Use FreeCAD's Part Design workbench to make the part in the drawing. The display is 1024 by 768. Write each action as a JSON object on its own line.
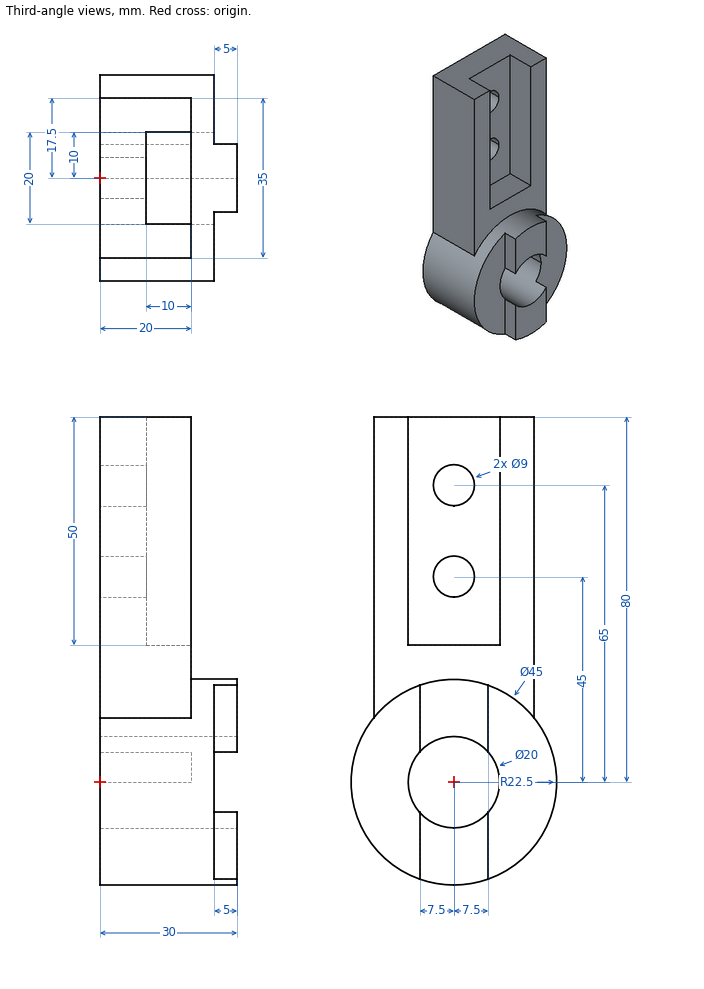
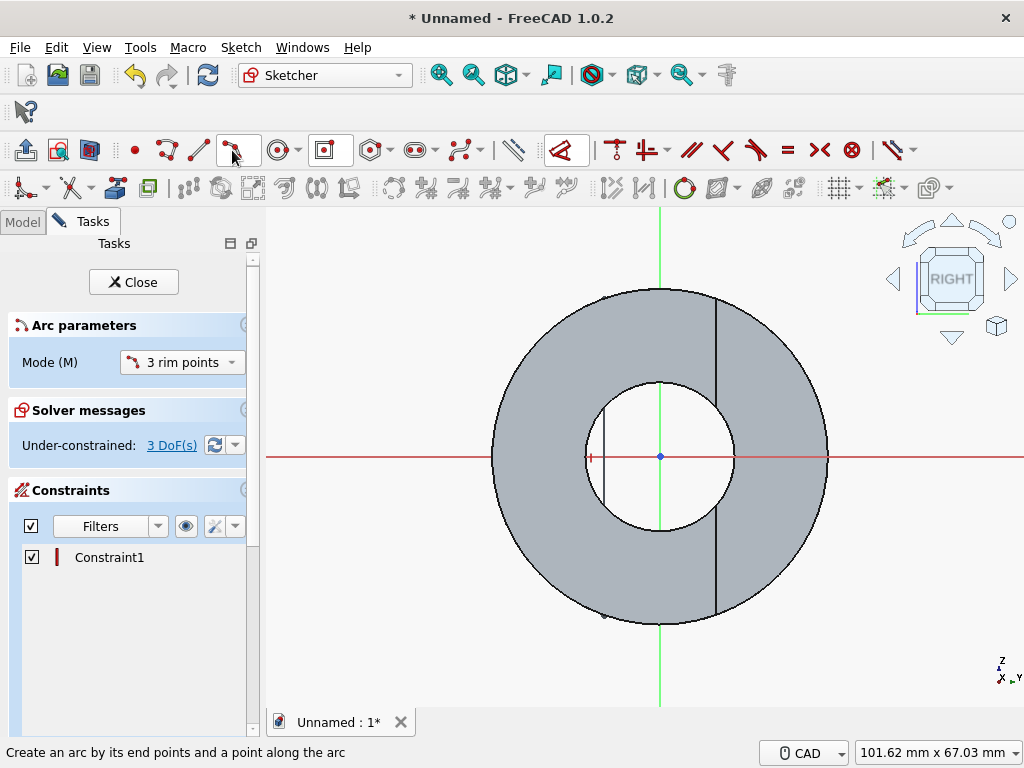
{"action": "left_click", "coordinate": [604, 300]}
{"action": "left_click", "coordinate": [604, 616]}
{"action": "left_click", "coordinate": [497, 416]}
{"action": "key", "text": "Escape"}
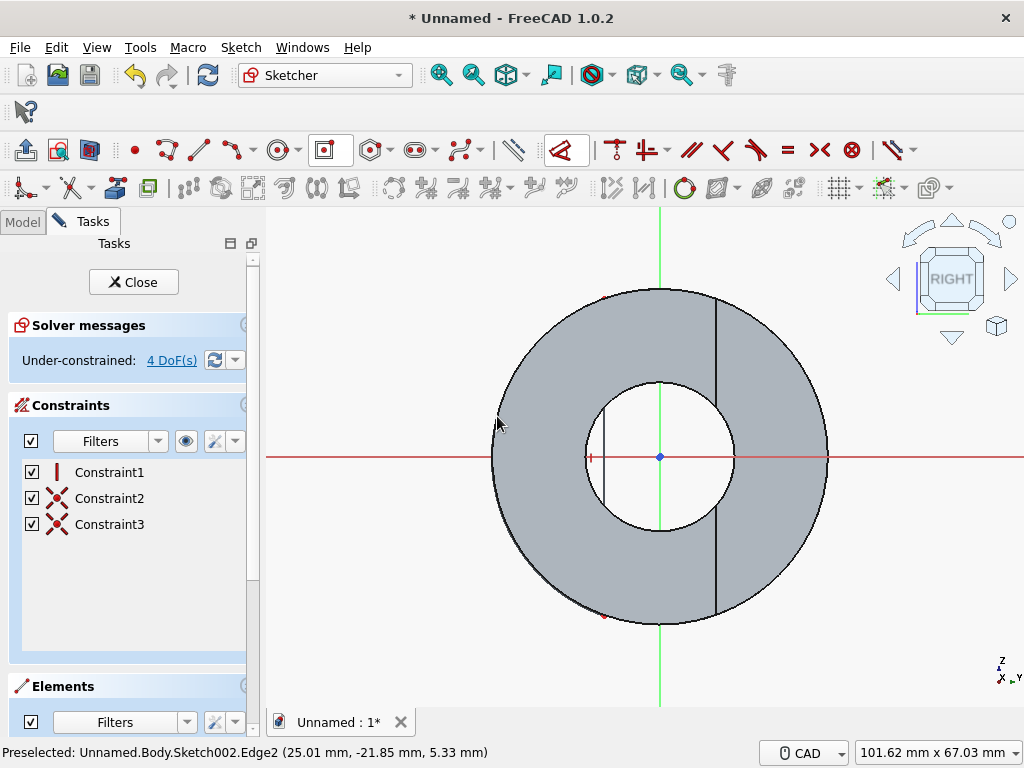
{"action": "left_click_drag", "start_coordinate": [649, 447], "coordinate": [670, 468]}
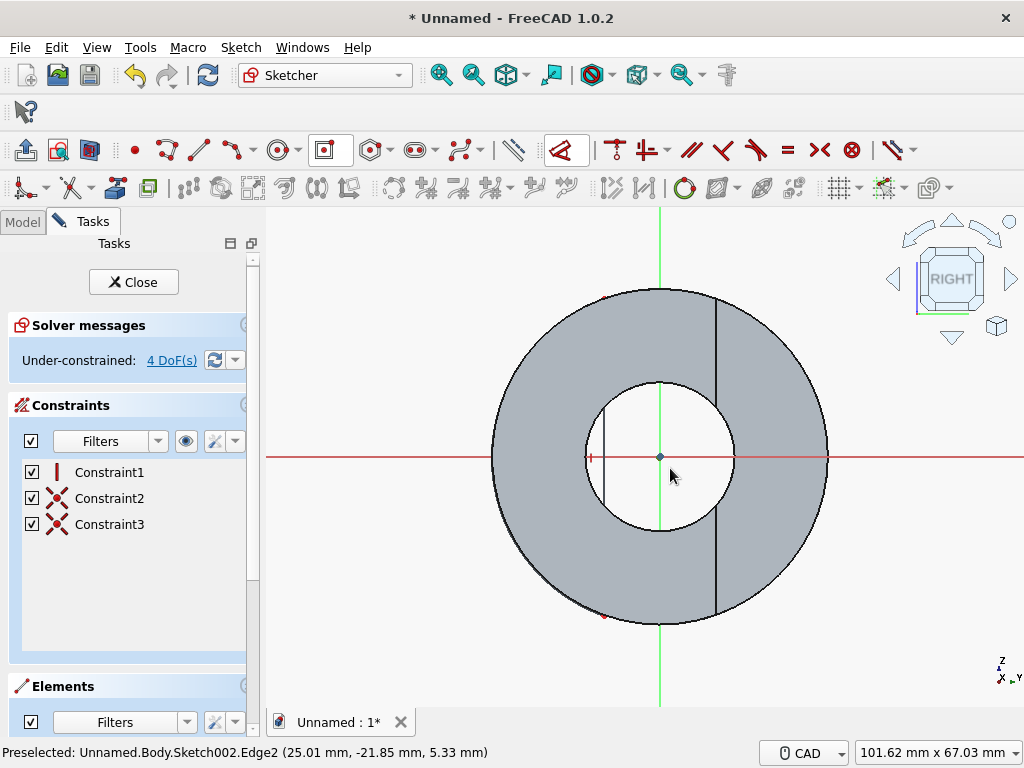
{"action": "left_click", "coordinate": [616, 150]}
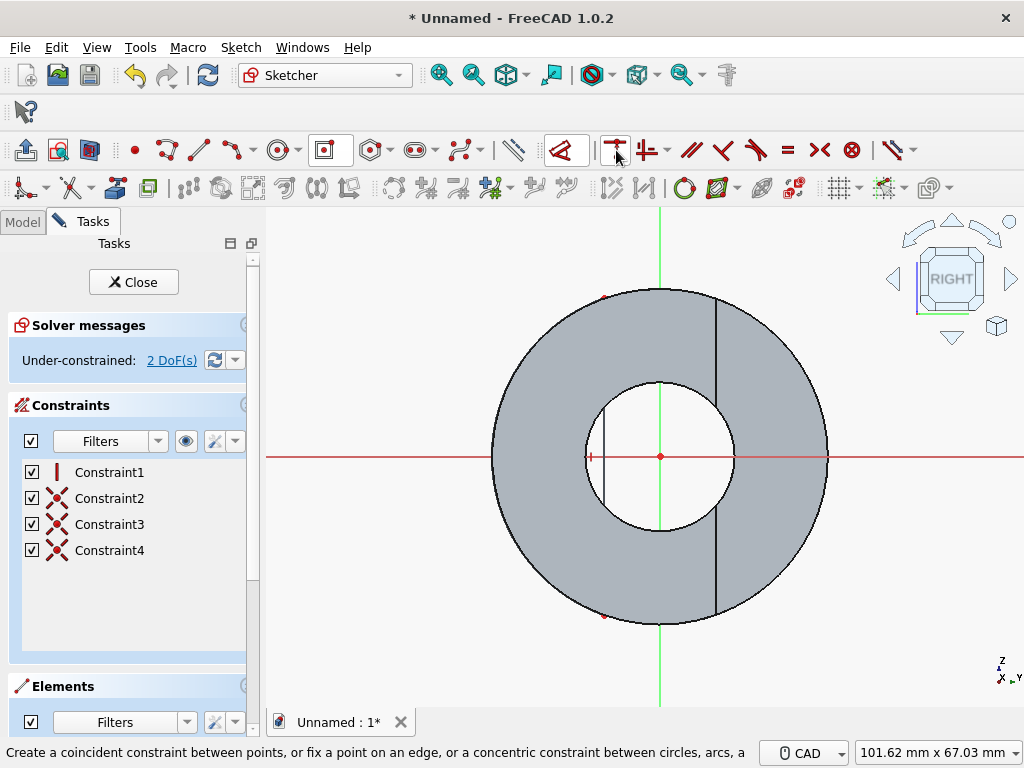
{"action": "left_click", "coordinate": [512, 377]}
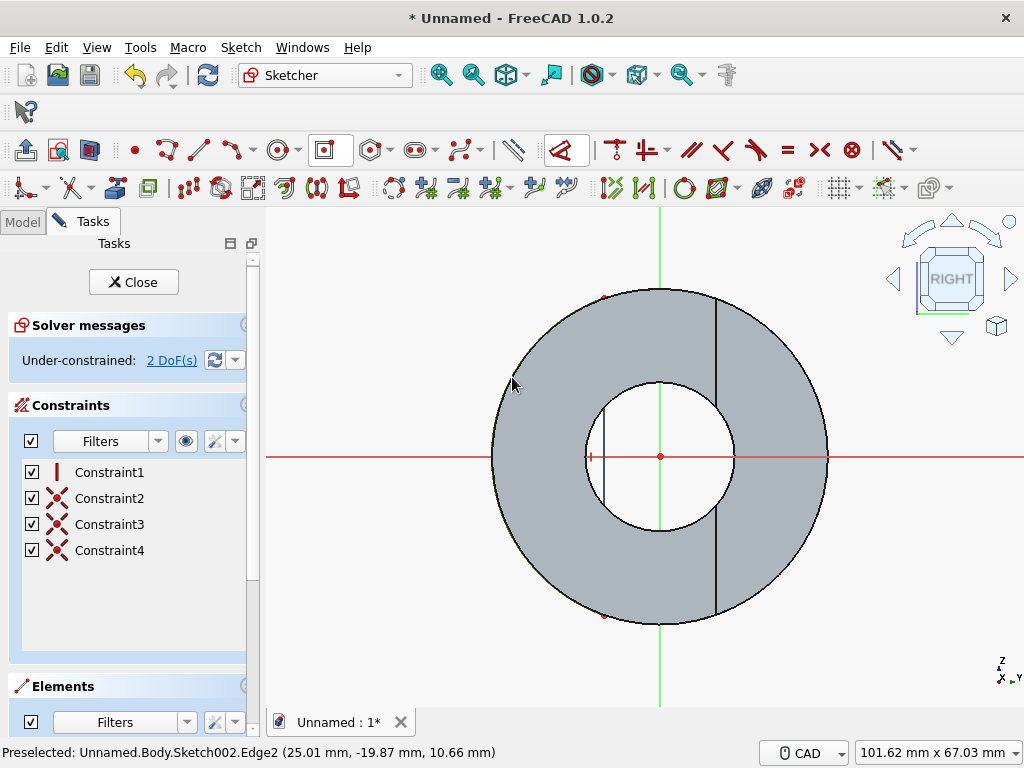
{"action": "key", "text": "k r"}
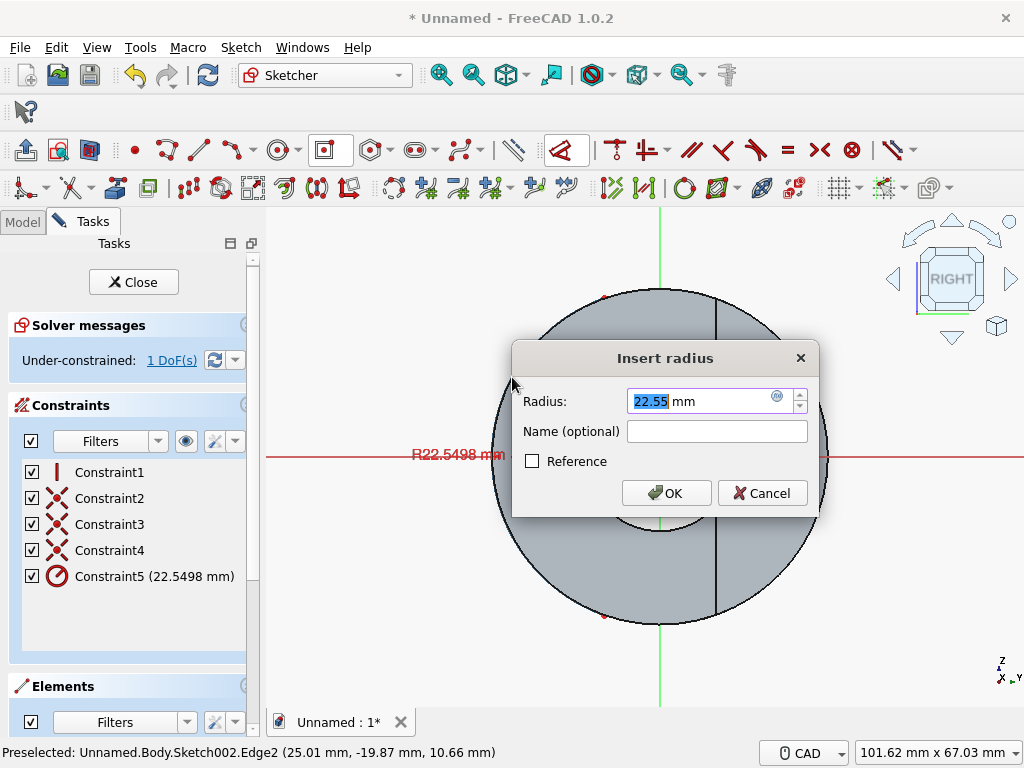
{"action": "type", "text": "22.5"}
{"action": "key", "text": "Return"}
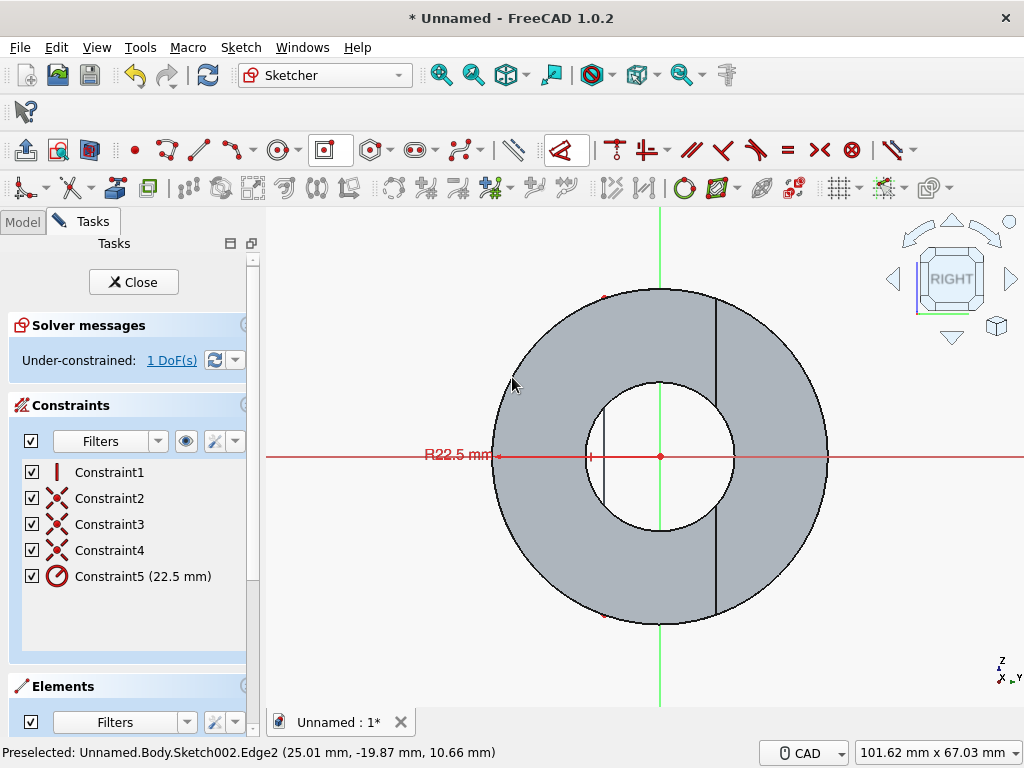
{"action": "left_click", "coordinate": [604, 615]}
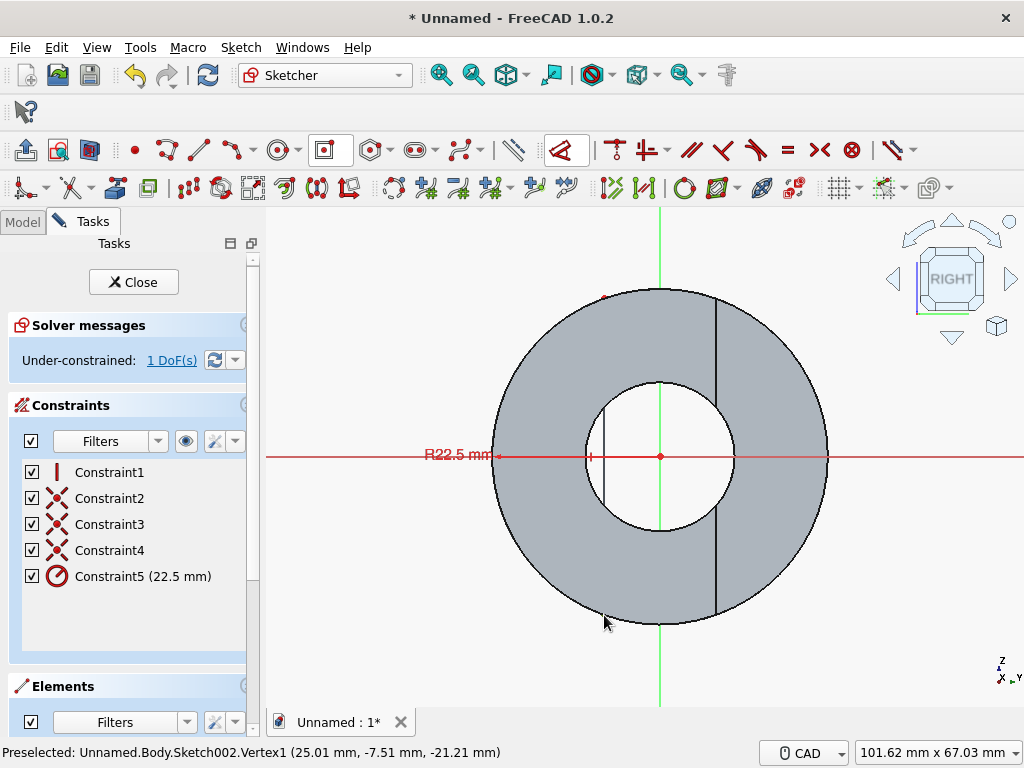
{"action": "left_click", "coordinate": [584, 150]}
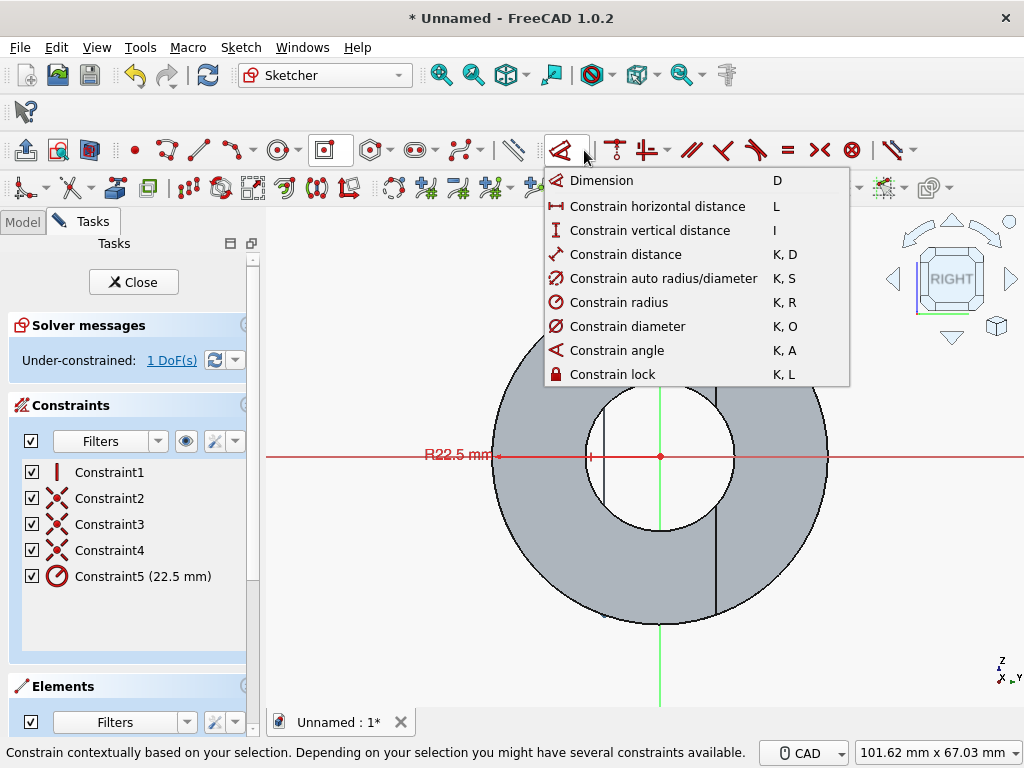
{"action": "left_click", "coordinate": [697, 206]}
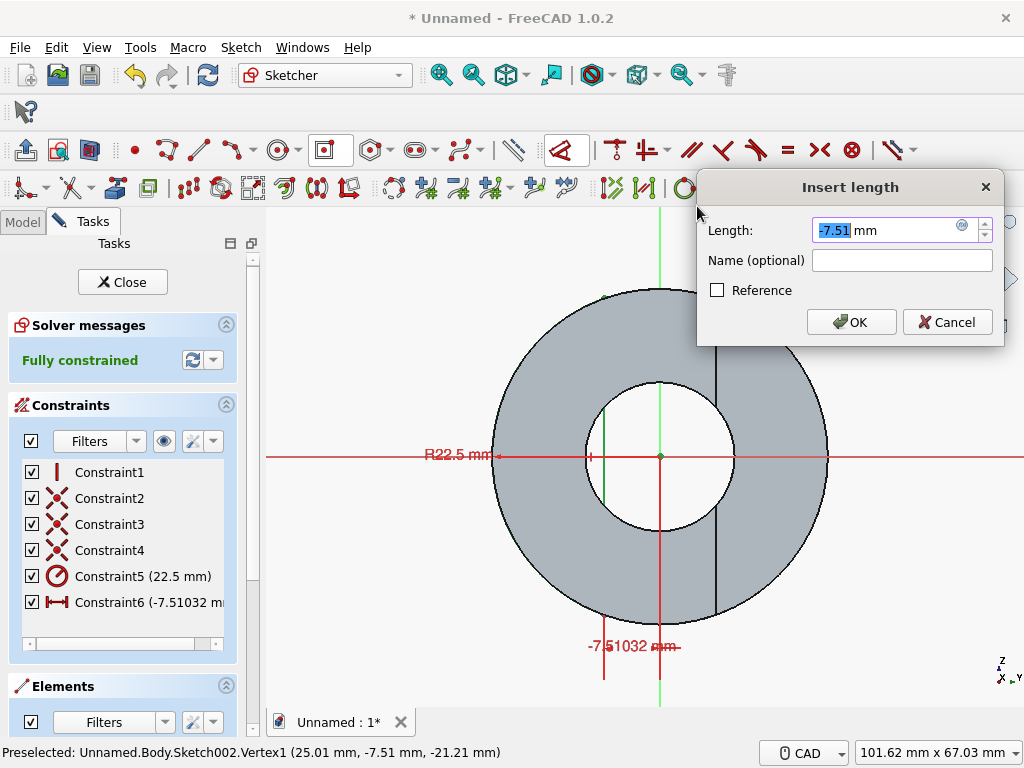
{"action": "type", "text": "-7.5"}
{"action": "key", "text": "Return"}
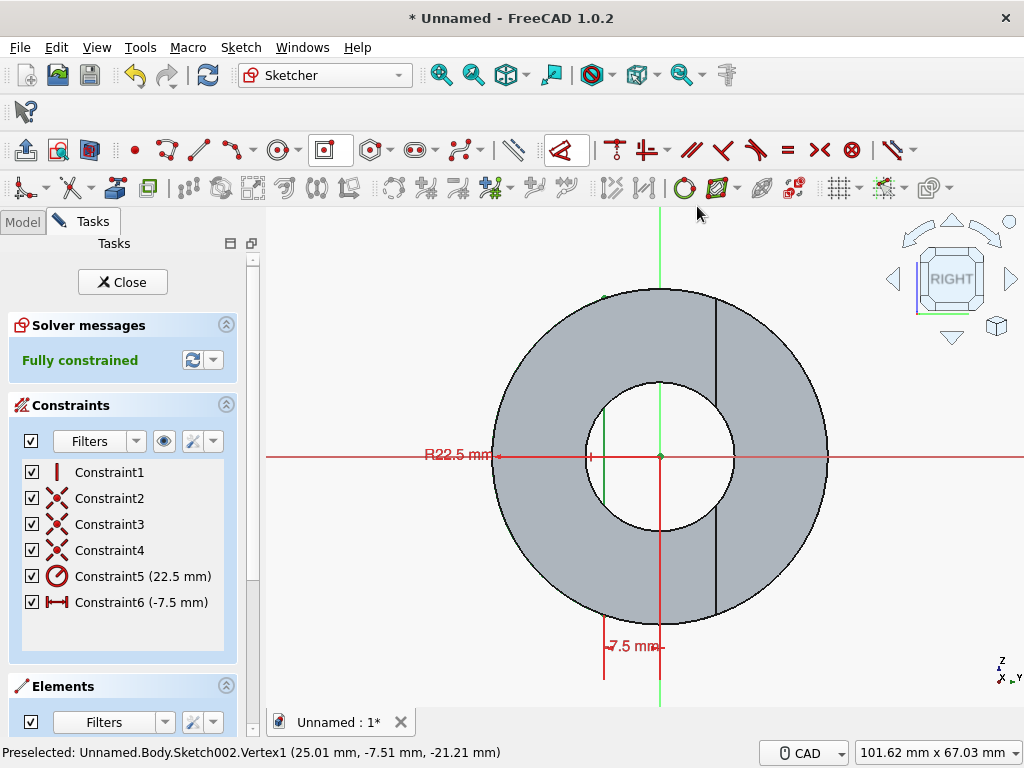
{"action": "left_click", "coordinate": [123, 282]}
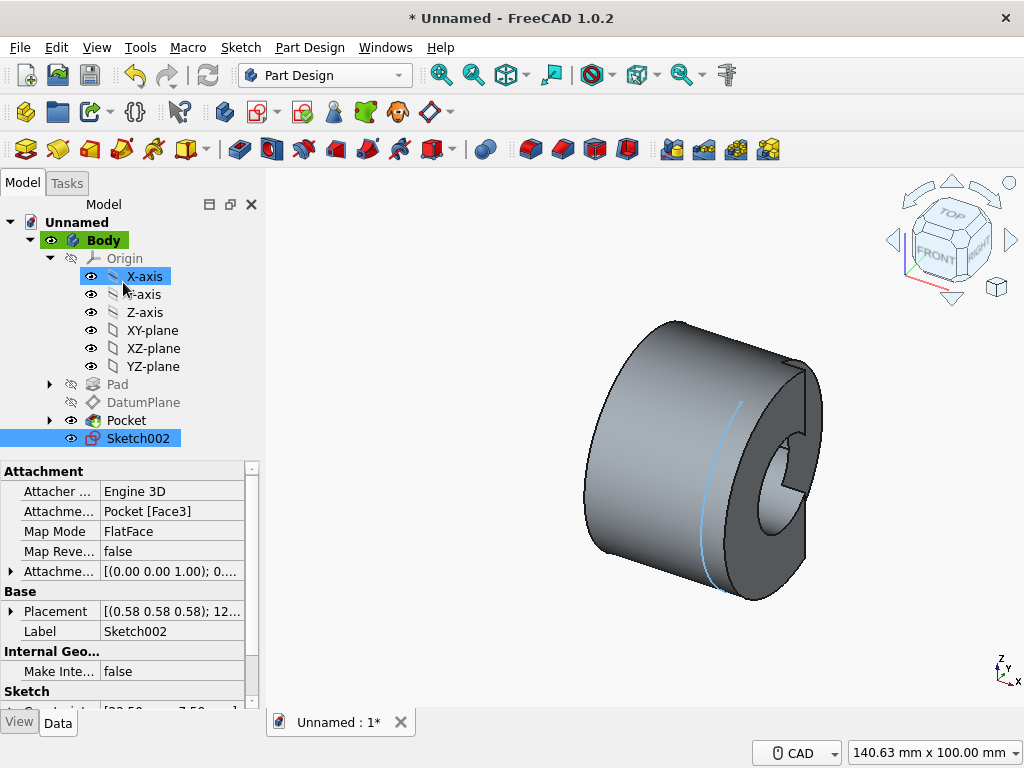
{"action": "left_click", "coordinate": [240, 150]}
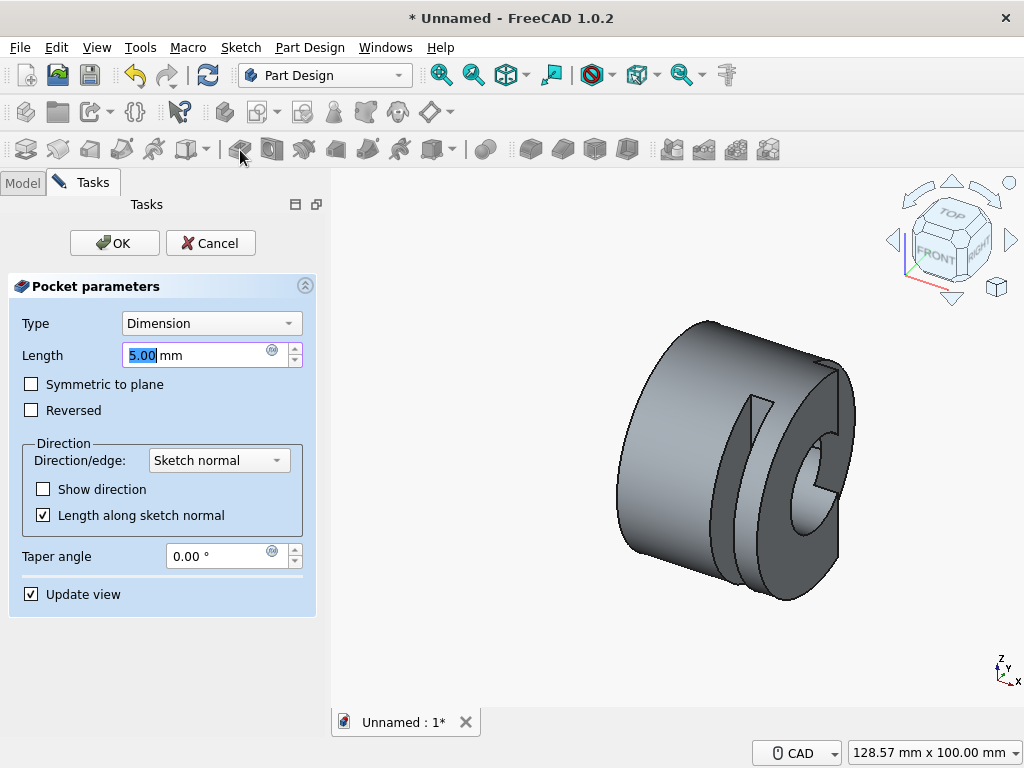
{"action": "type", "text": "5"}
{"action": "key", "text": "Tab"}